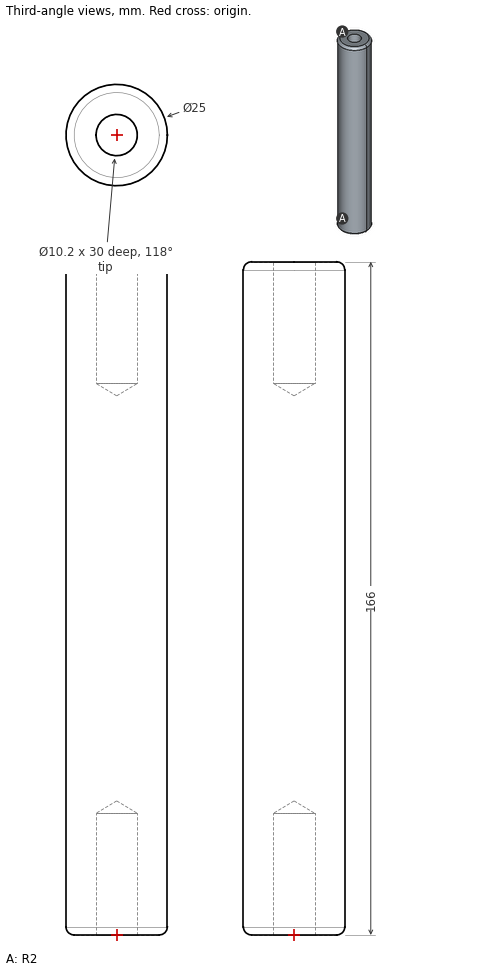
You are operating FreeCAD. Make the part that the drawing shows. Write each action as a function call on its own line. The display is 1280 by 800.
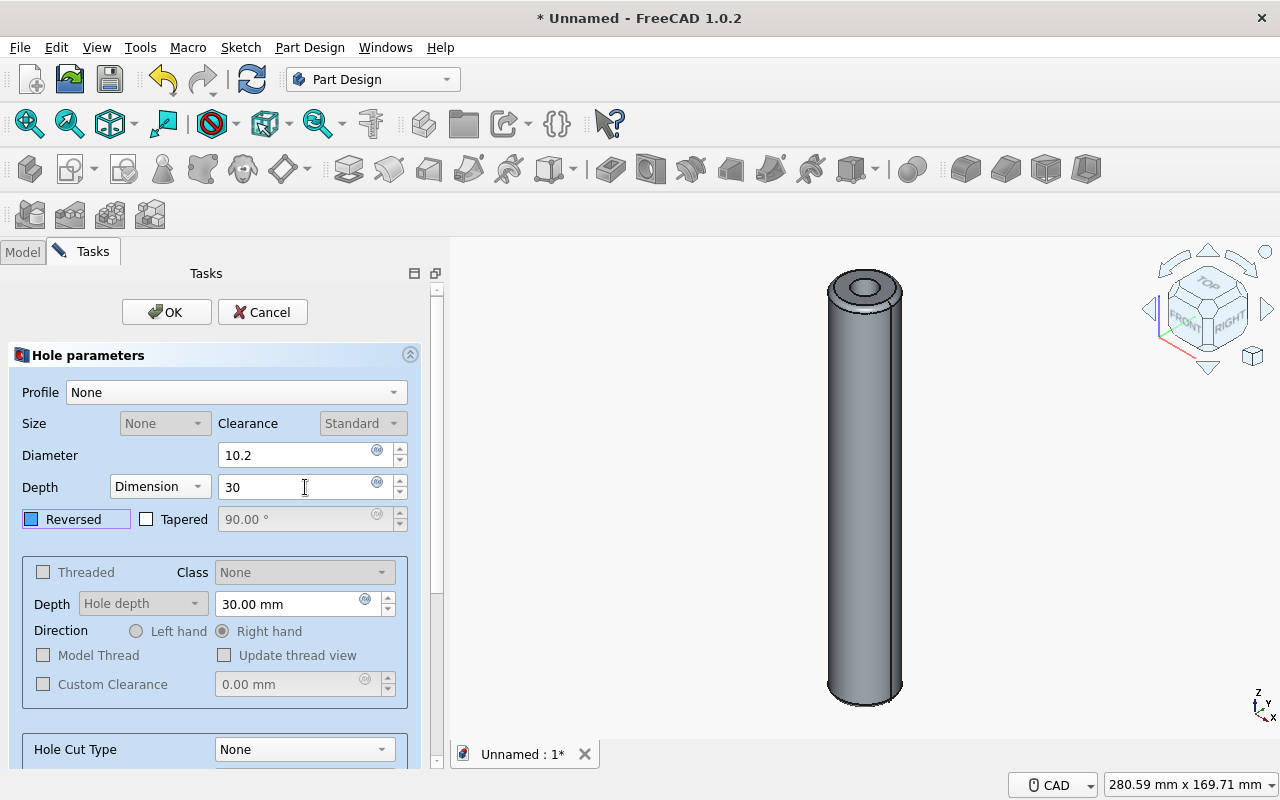
click(30, 519)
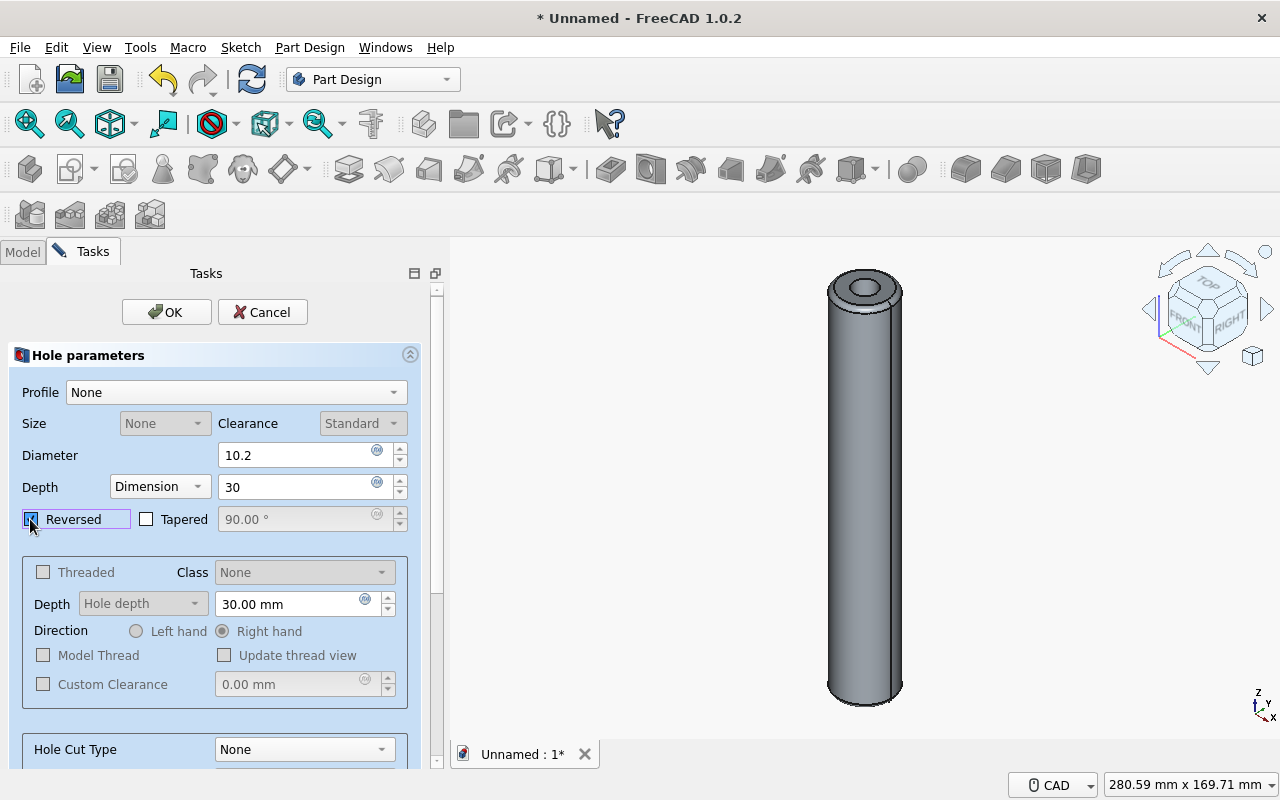
click(167, 312)